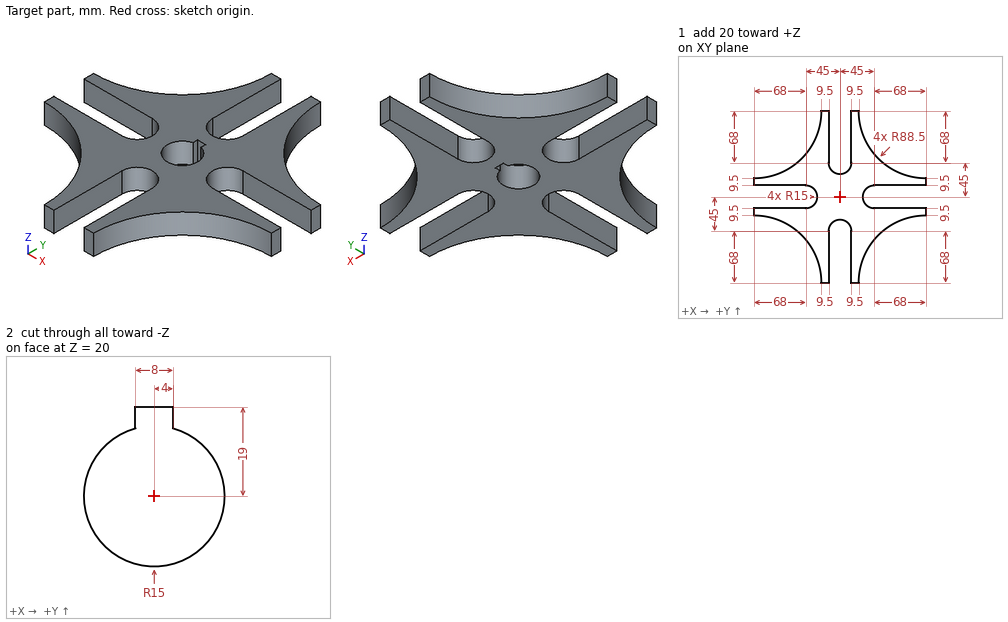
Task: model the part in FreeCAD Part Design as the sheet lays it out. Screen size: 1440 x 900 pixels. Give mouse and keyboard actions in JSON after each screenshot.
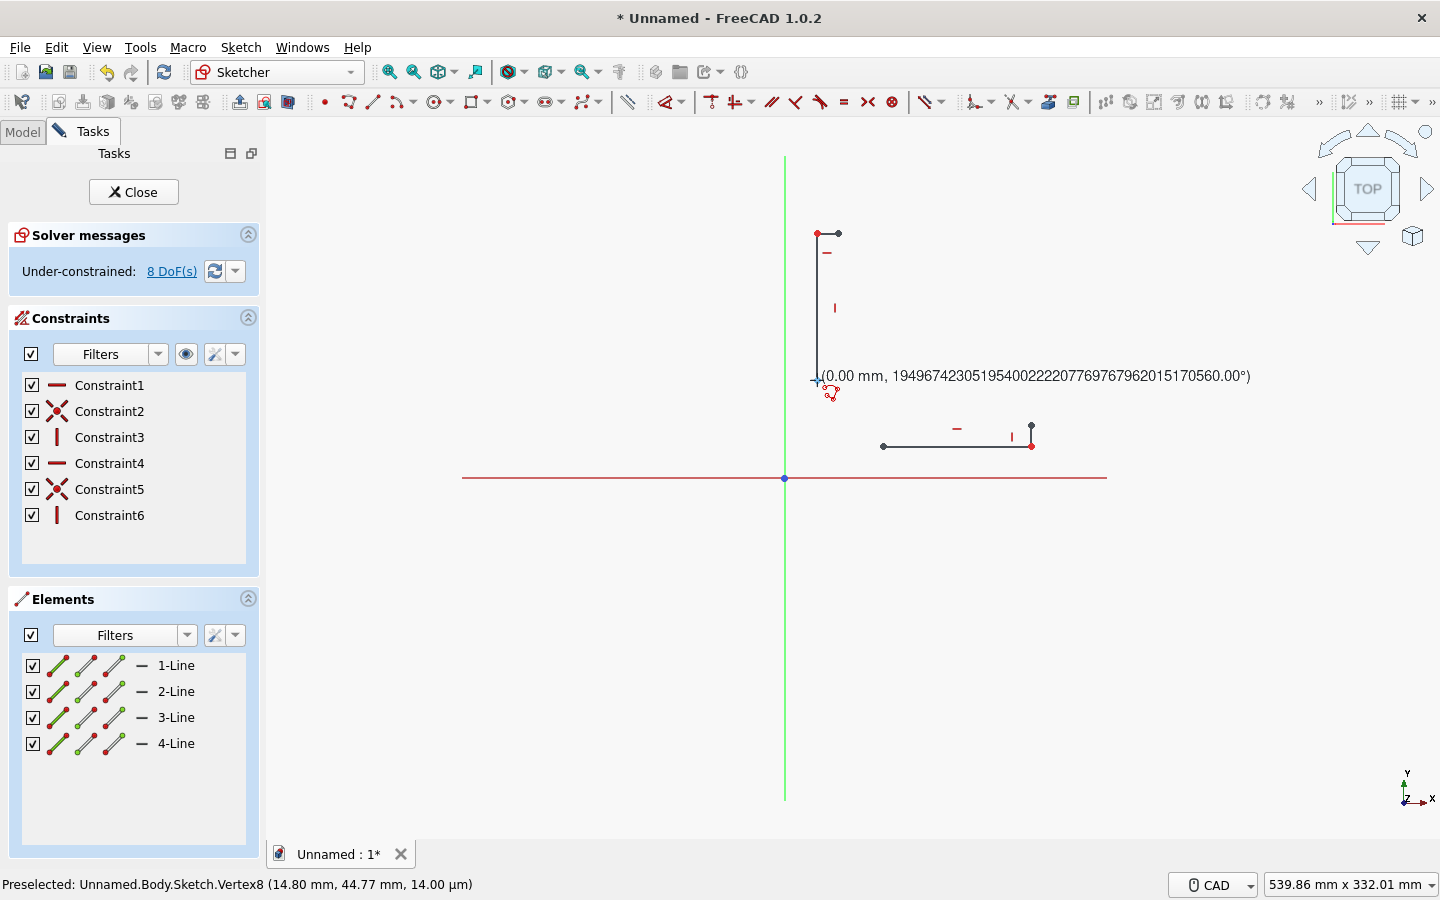
{"action": "left_click", "coordinate": [752, 380]}
{"action": "left_click", "coordinate": [752, 233]}
{"action": "left_click", "coordinate": [732, 233]}
{"action": "right_click", "coordinate": [732, 233]}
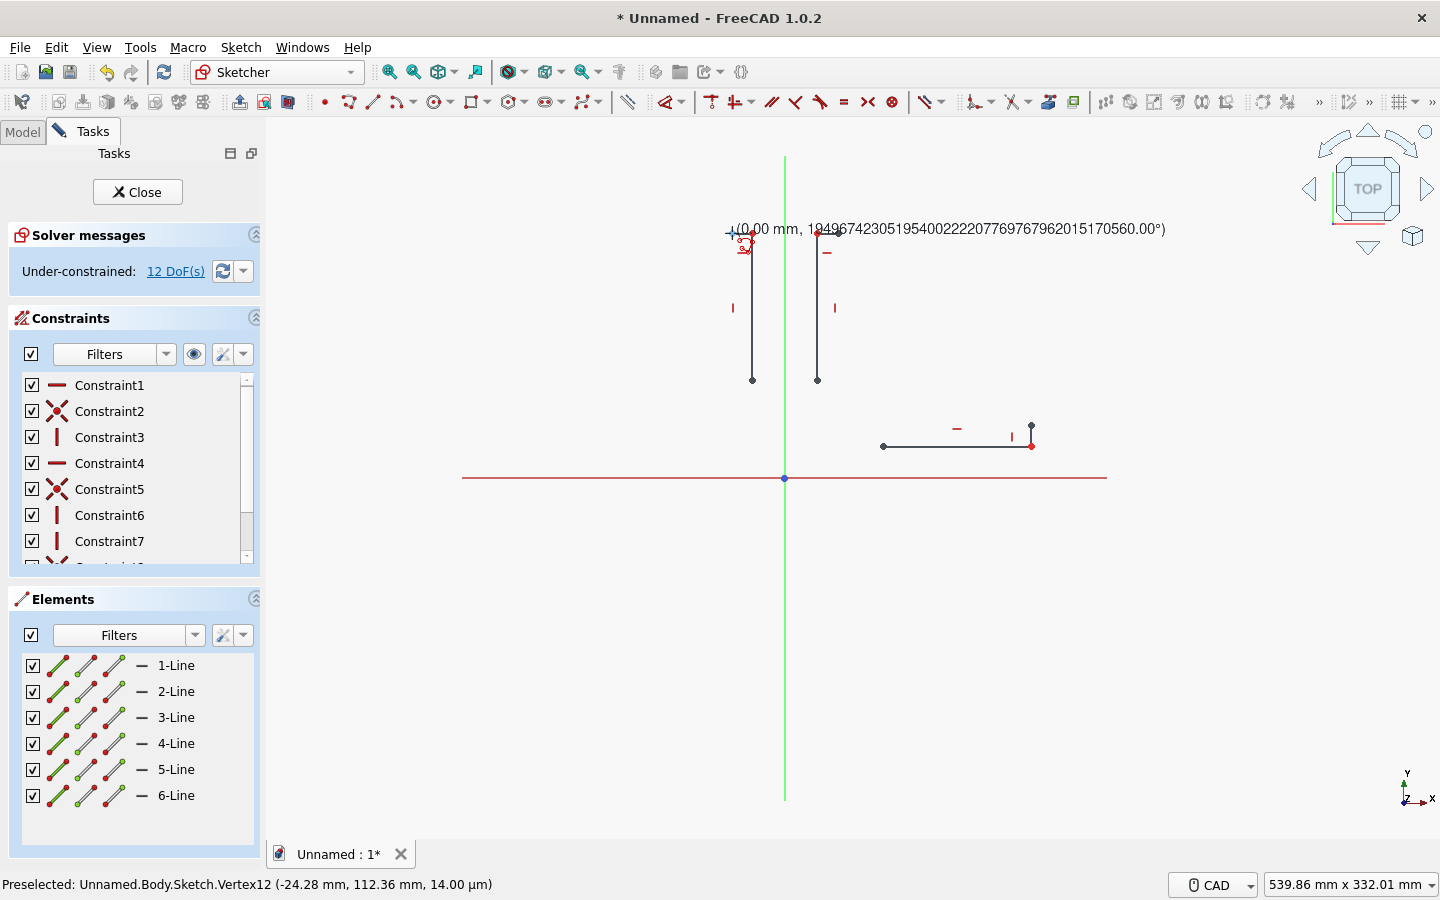
{"action": "left_click", "coordinate": [539, 425]}
{"action": "left_click", "coordinate": [539, 446]}
{"action": "left_click", "coordinate": [687, 446]}
{"action": "right_click", "coordinate": [687, 446]}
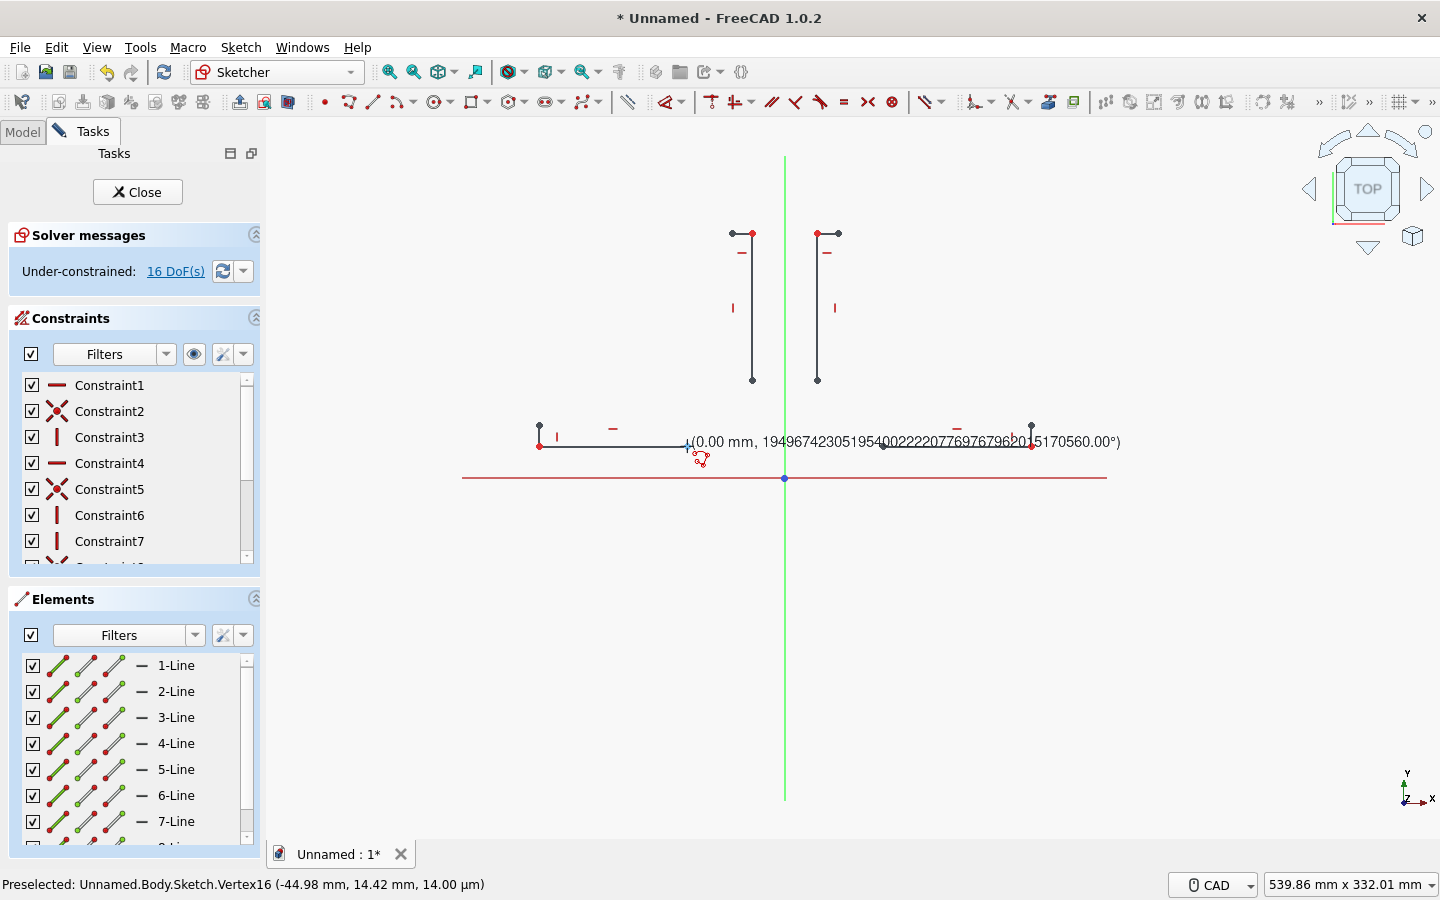
{"action": "left_click", "coordinate": [687, 511]}
{"action": "left_click", "coordinate": [539, 511]}
{"action": "left_click", "coordinate": [539, 532]}
{"action": "right_click", "coordinate": [539, 532]}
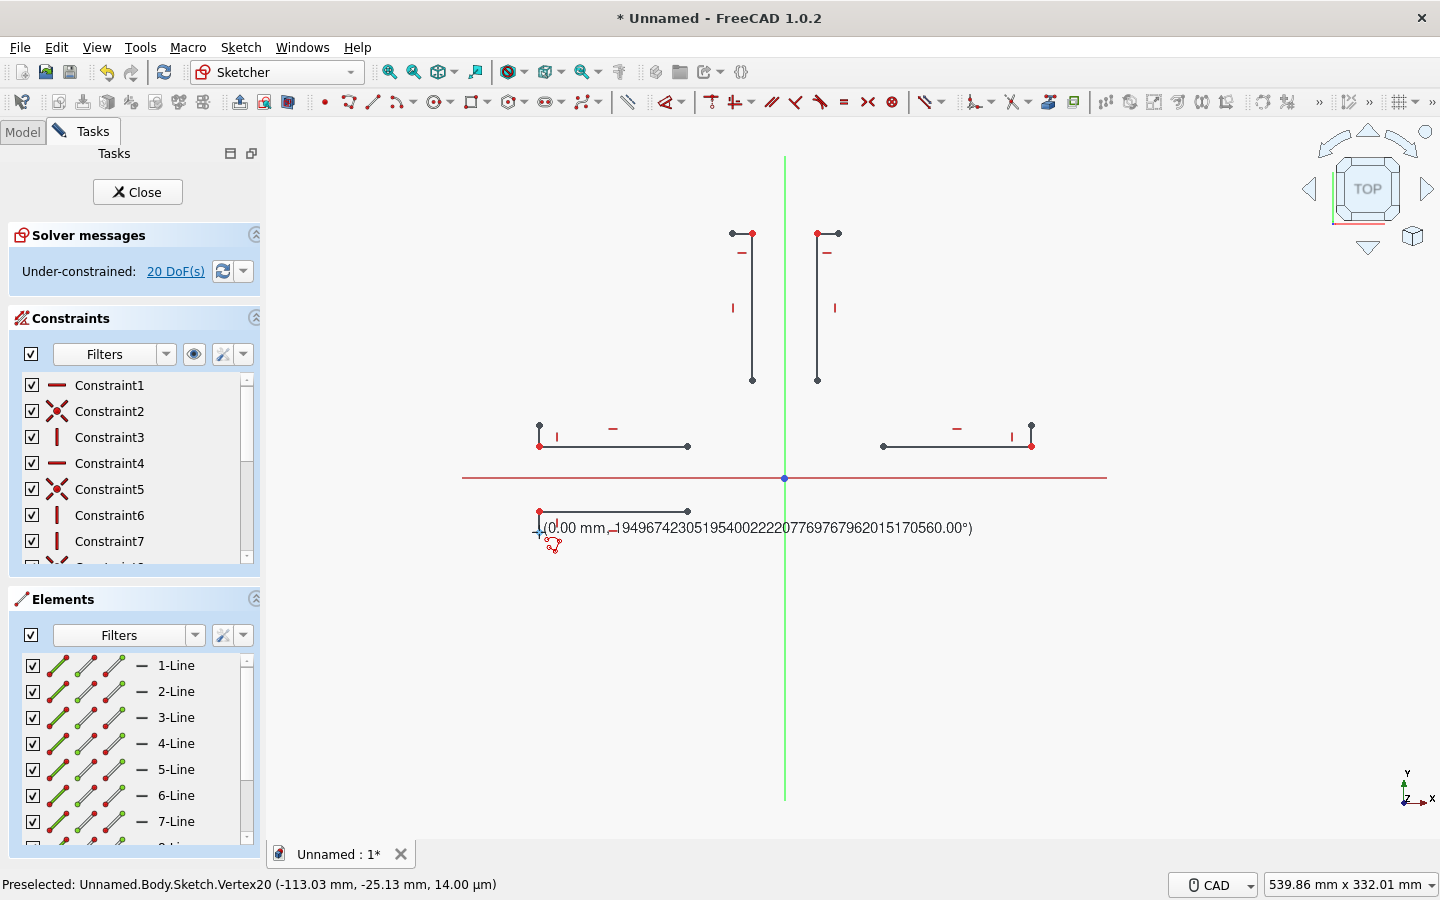
{"action": "left_click", "coordinate": [732, 724]}
{"action": "left_click", "coordinate": [752, 724]}
{"action": "left_click", "coordinate": [752, 576]}
{"action": "right_click", "coordinate": [752, 576]}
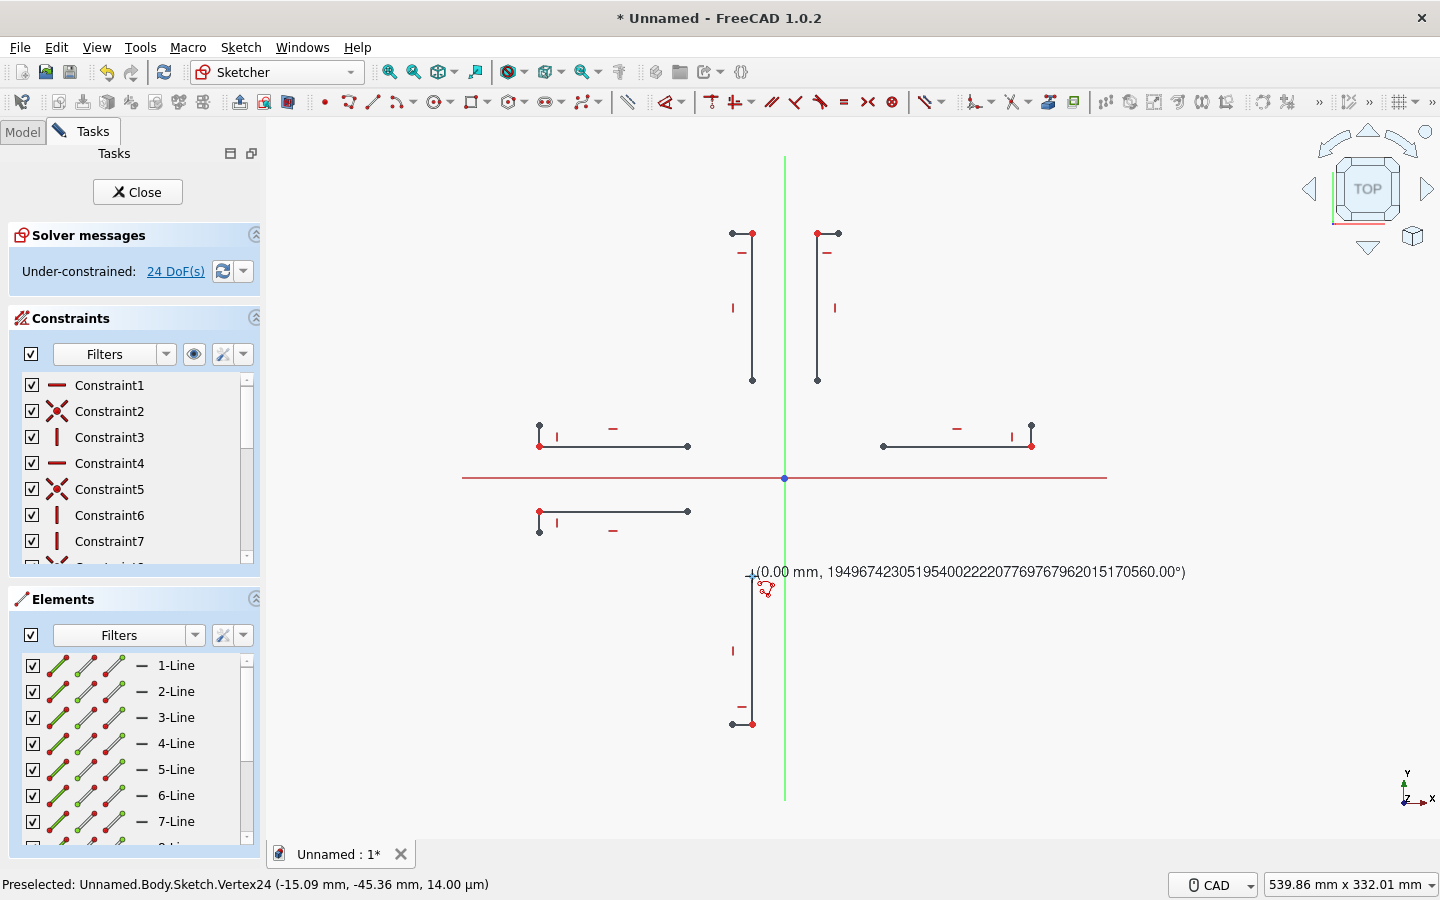
{"action": "left_click", "coordinate": [817, 576]}
{"action": "left_click", "coordinate": [817, 724]}
{"action": "left_click", "coordinate": [838, 724]}
{"action": "right_click", "coordinate": [838, 724]}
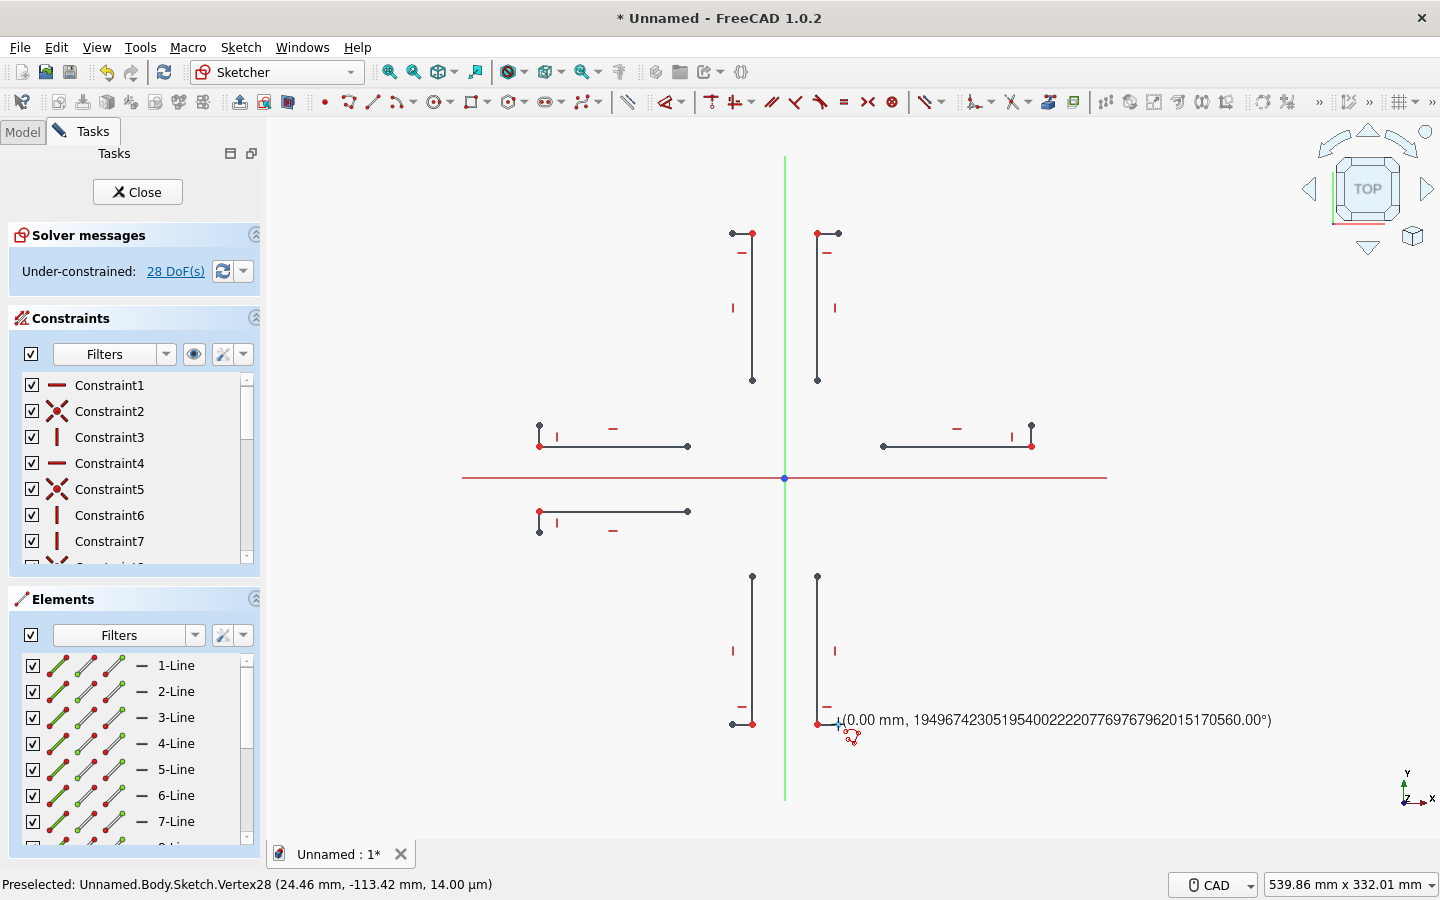
{"action": "left_click", "coordinate": [1031, 532]}
{"action": "left_click", "coordinate": [1031, 511]}
{"action": "left_click", "coordinate": [883, 511]}
{"action": "right_click", "coordinate": [883, 511]}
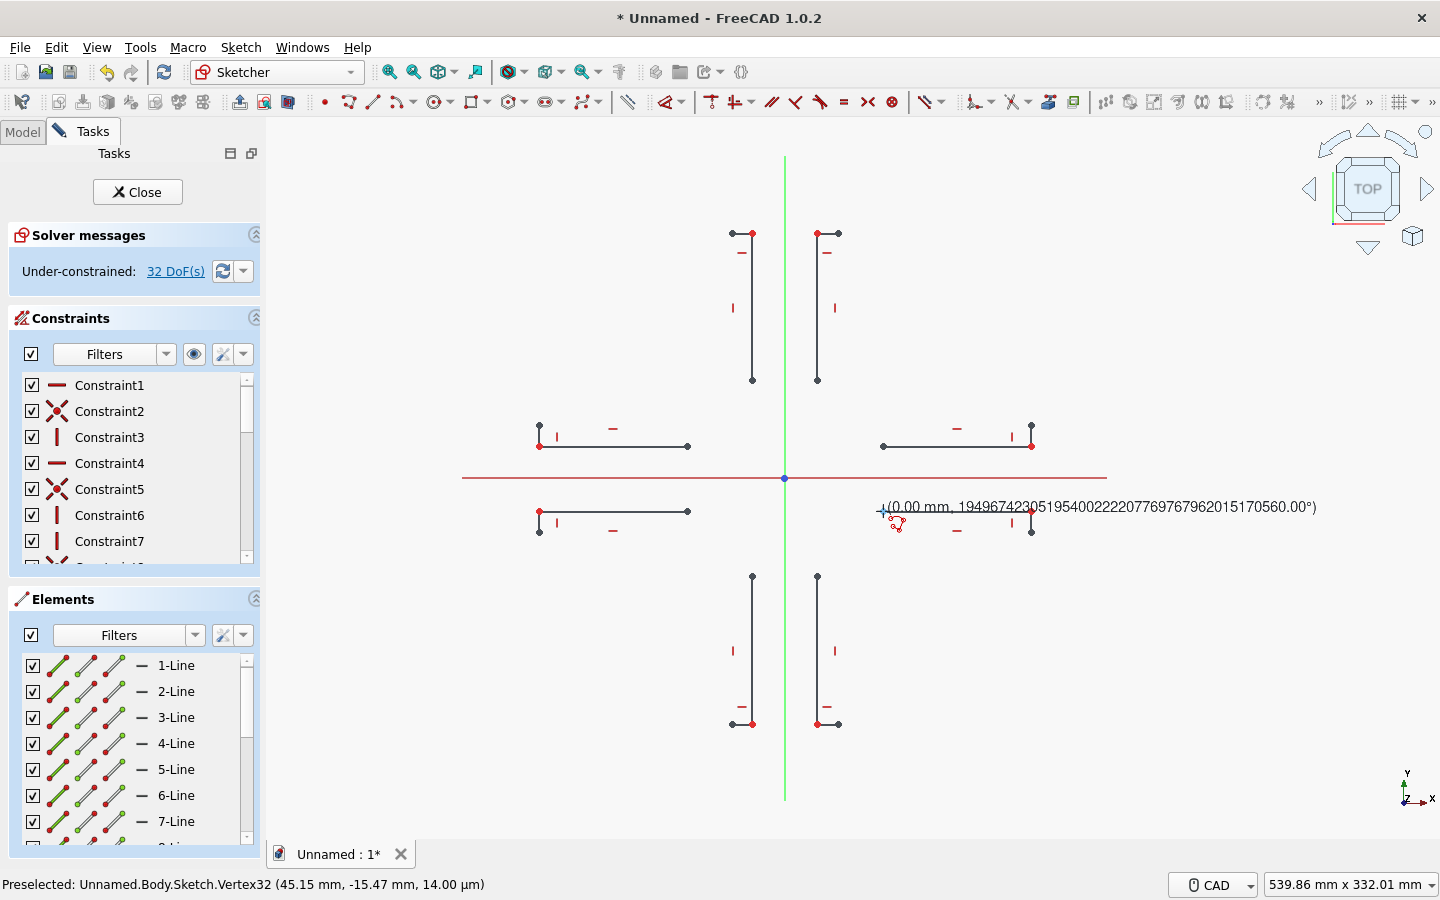
{"action": "left_click", "coordinate": [416, 102]}